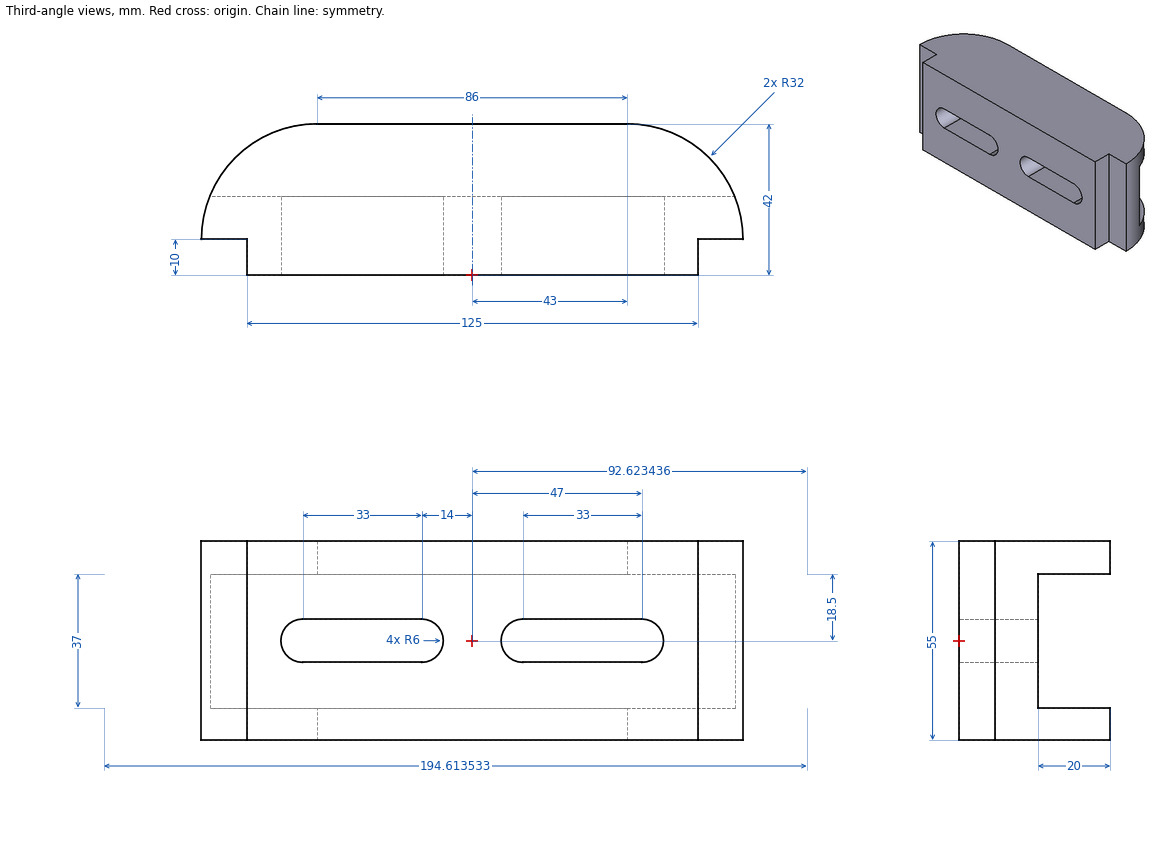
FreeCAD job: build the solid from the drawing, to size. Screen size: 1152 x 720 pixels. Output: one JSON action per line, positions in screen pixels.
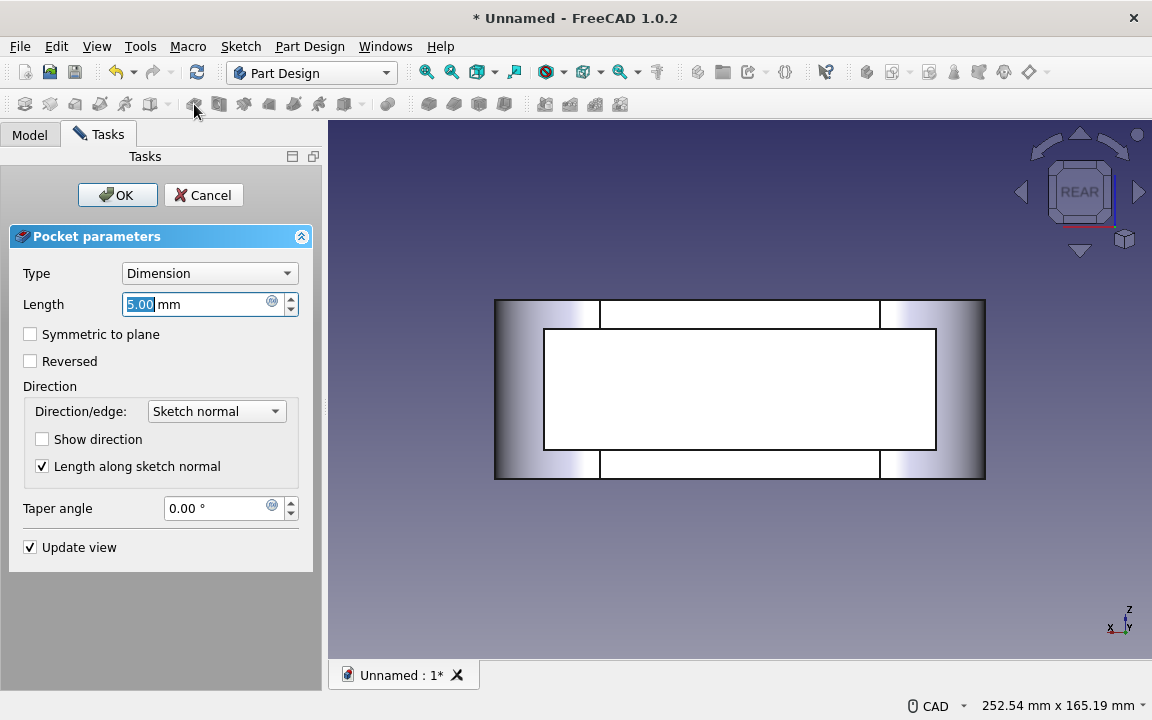
{"action": "type", "text": "20"}
{"action": "key", "text": "Tab"}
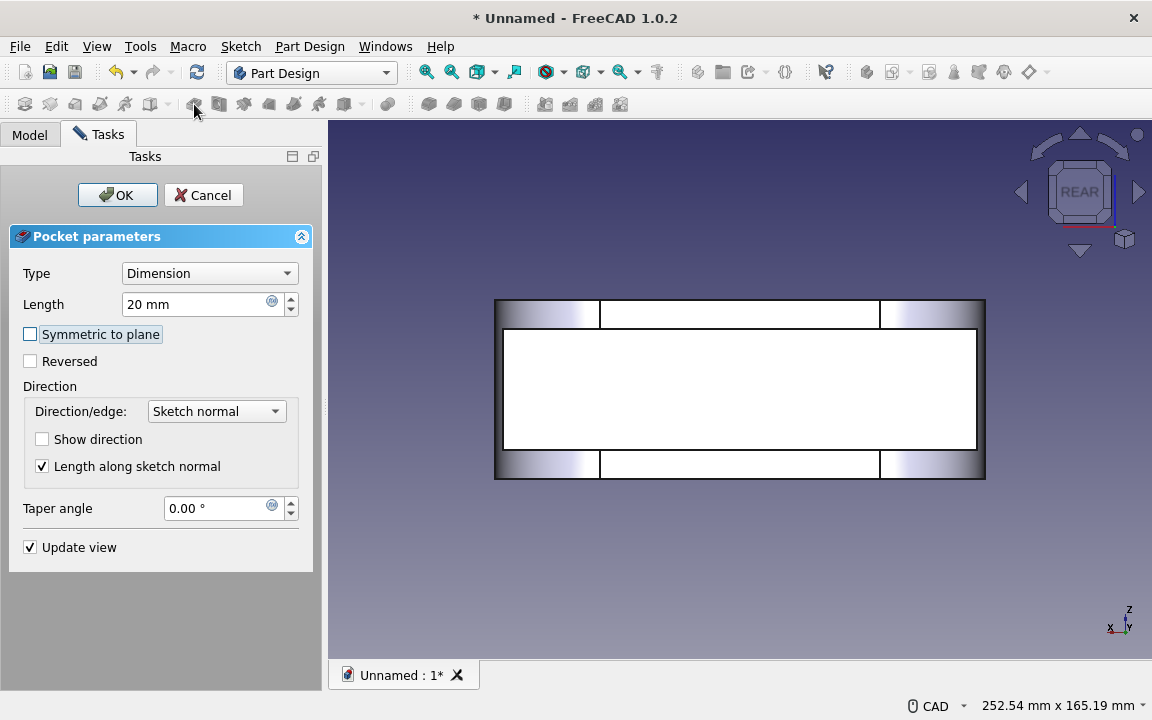
{"action": "left_click", "coordinate": [118, 195]}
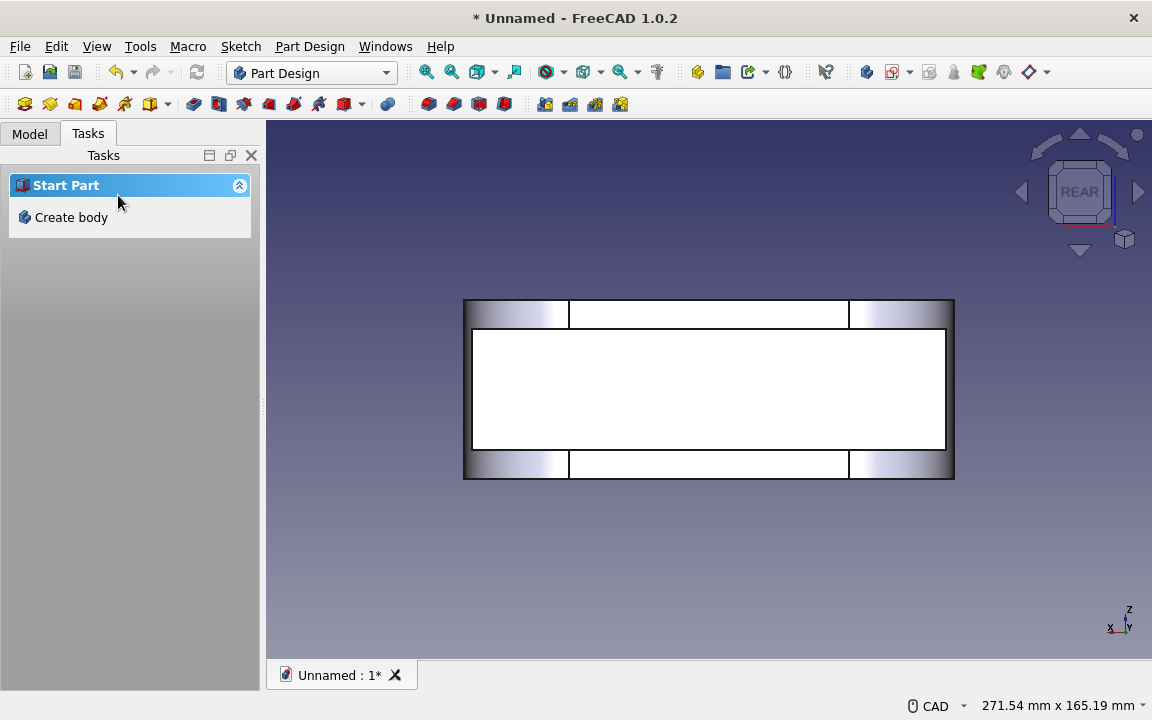
{"action": "left_click", "coordinate": [574, 388]}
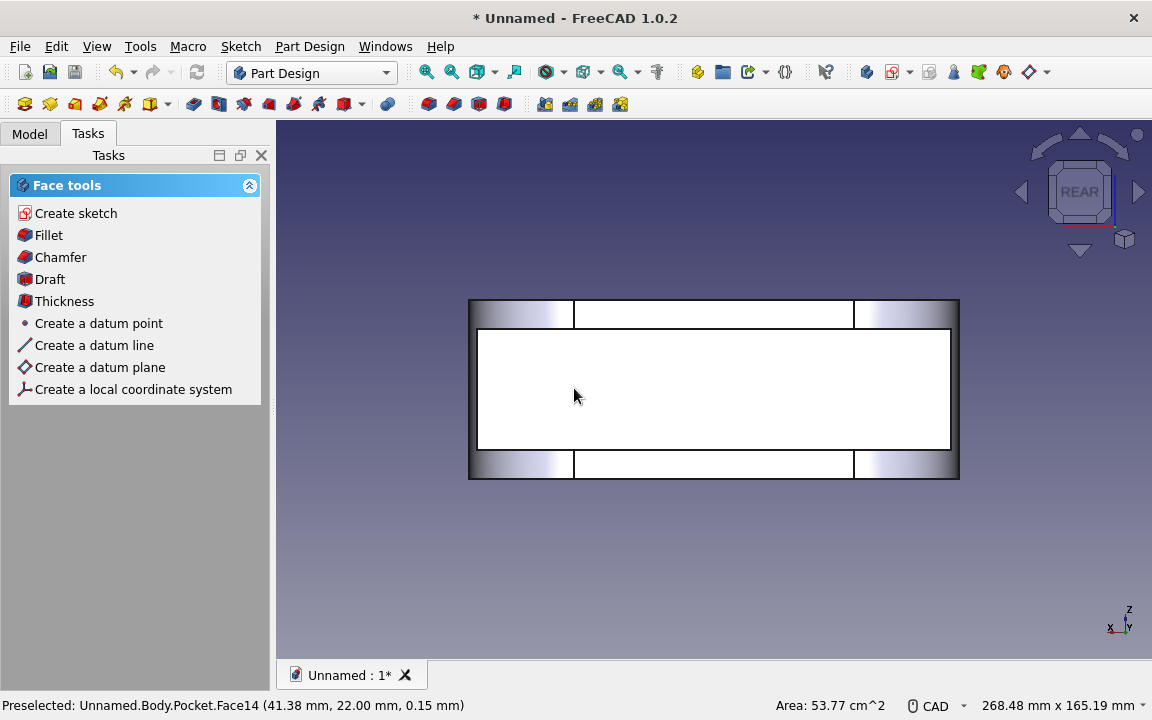
{"action": "left_click", "coordinate": [892, 72]}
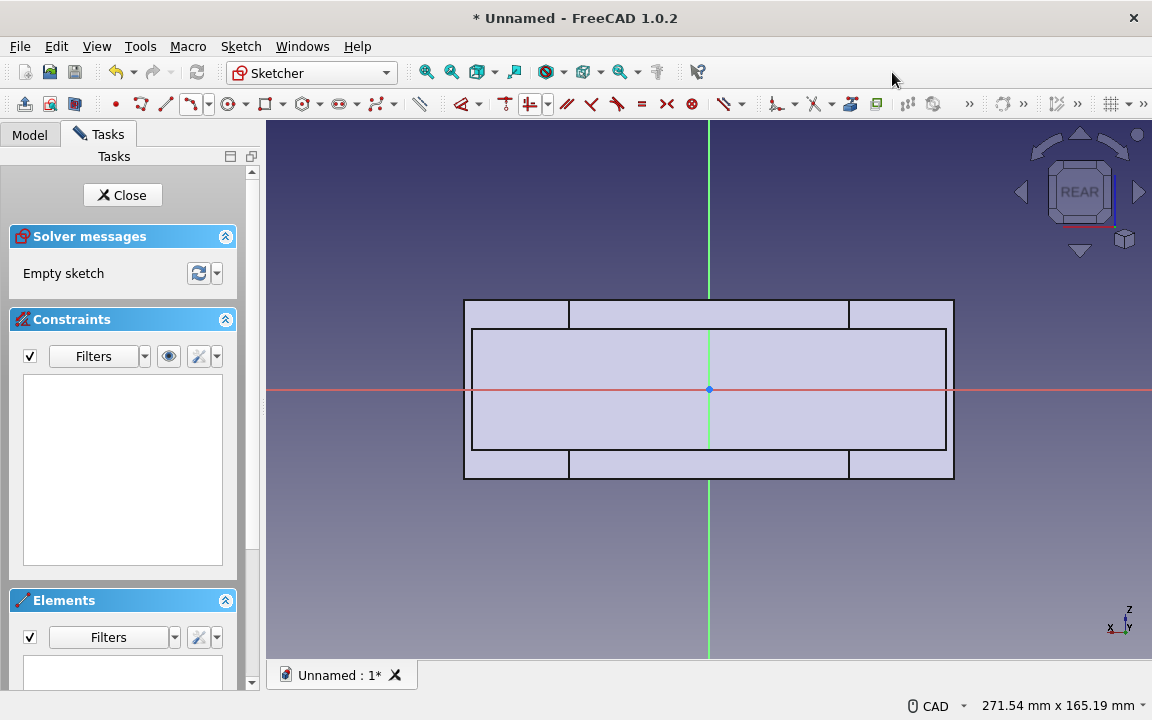
{"action": "left_click", "coordinate": [75, 104]}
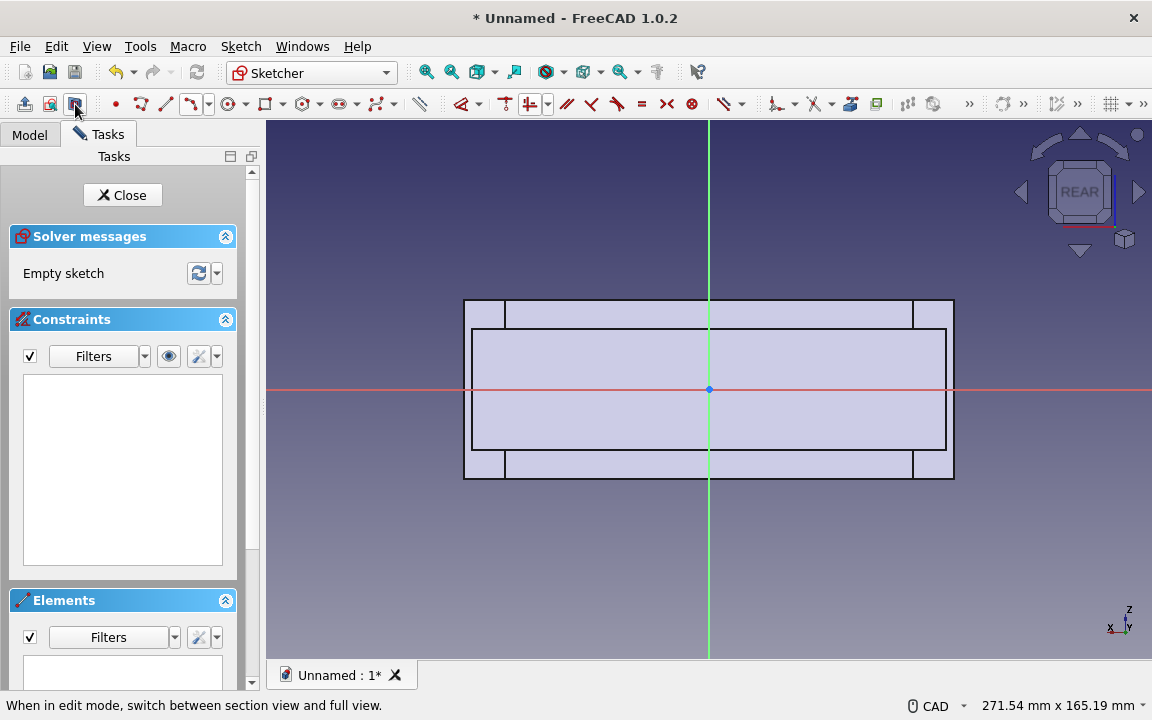
{"action": "scroll", "coordinate": [848, 390], "scroll_direction": "up", "scroll_amount": 2}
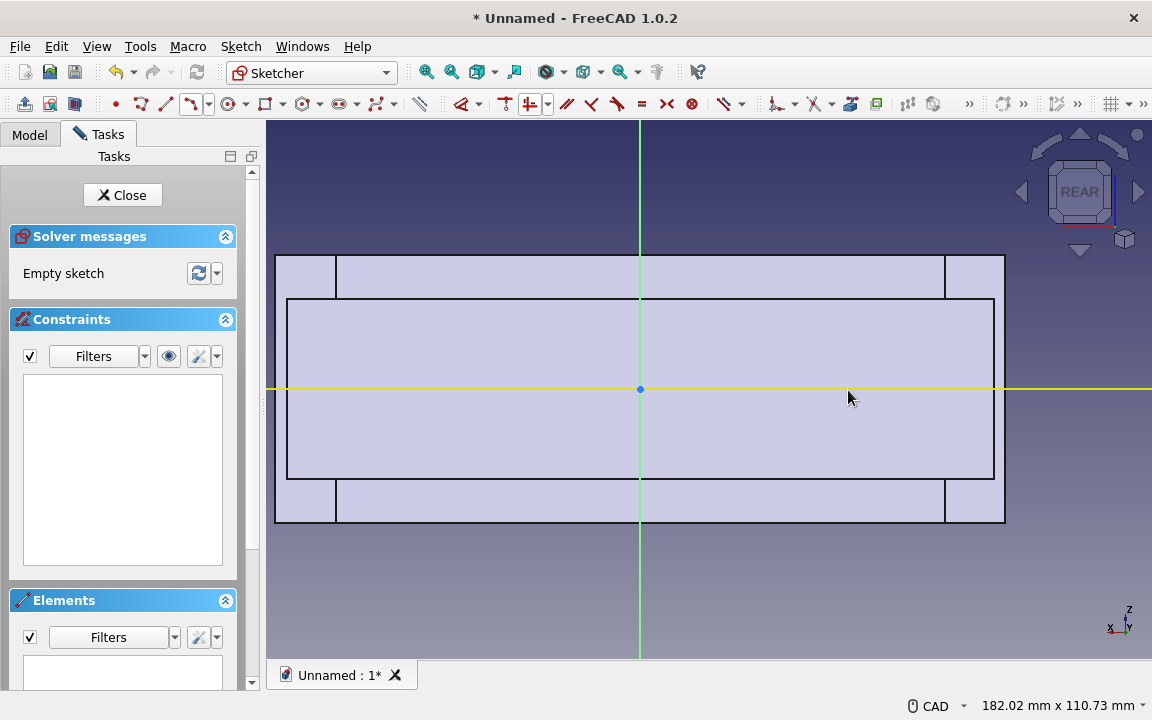
{"action": "left_click", "coordinate": [338, 104]}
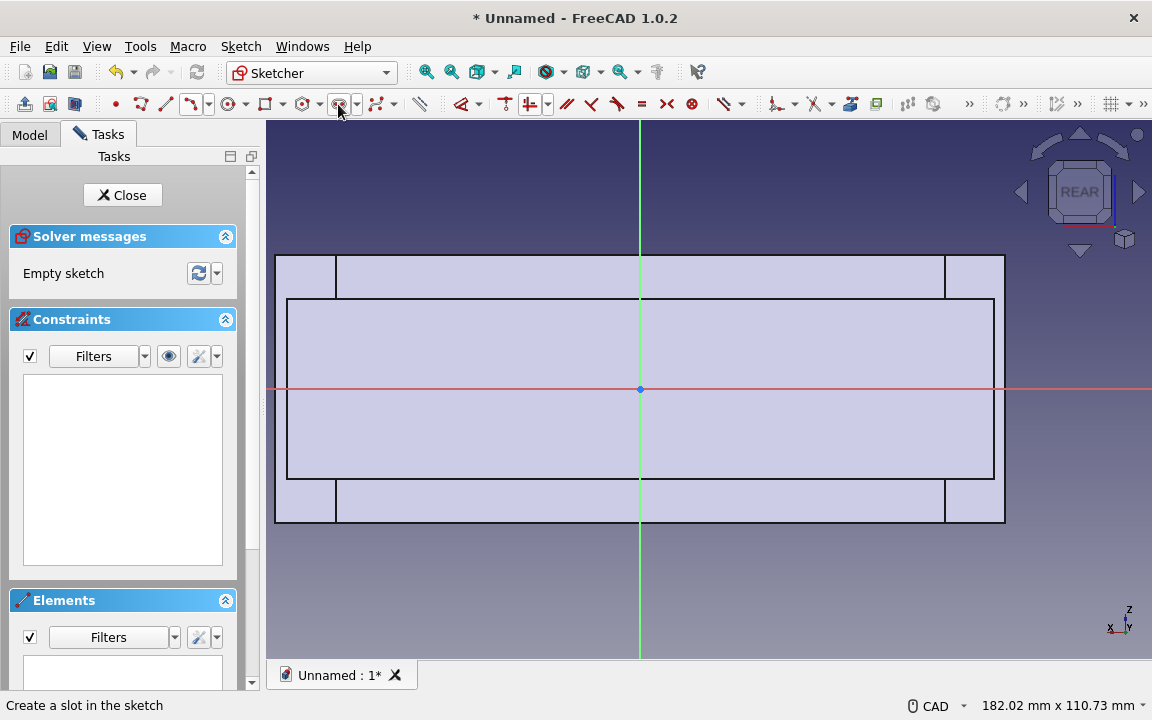
{"action": "left_click", "coordinate": [708, 389]}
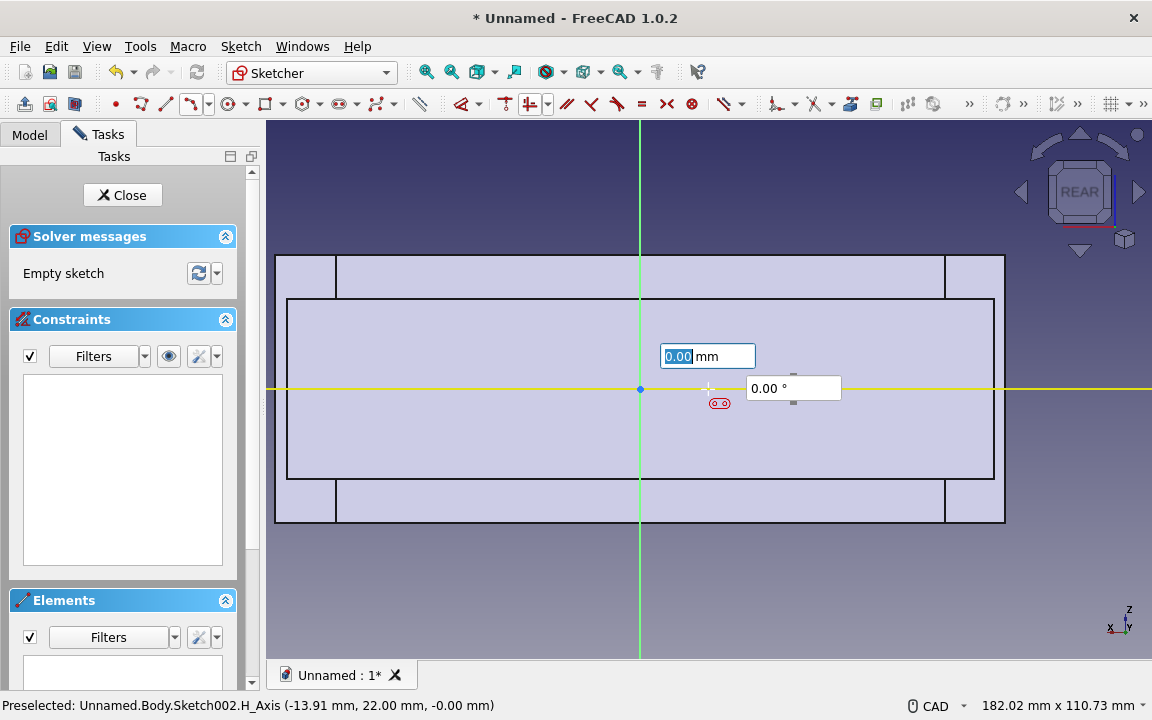
{"action": "left_click", "coordinate": [869, 380]}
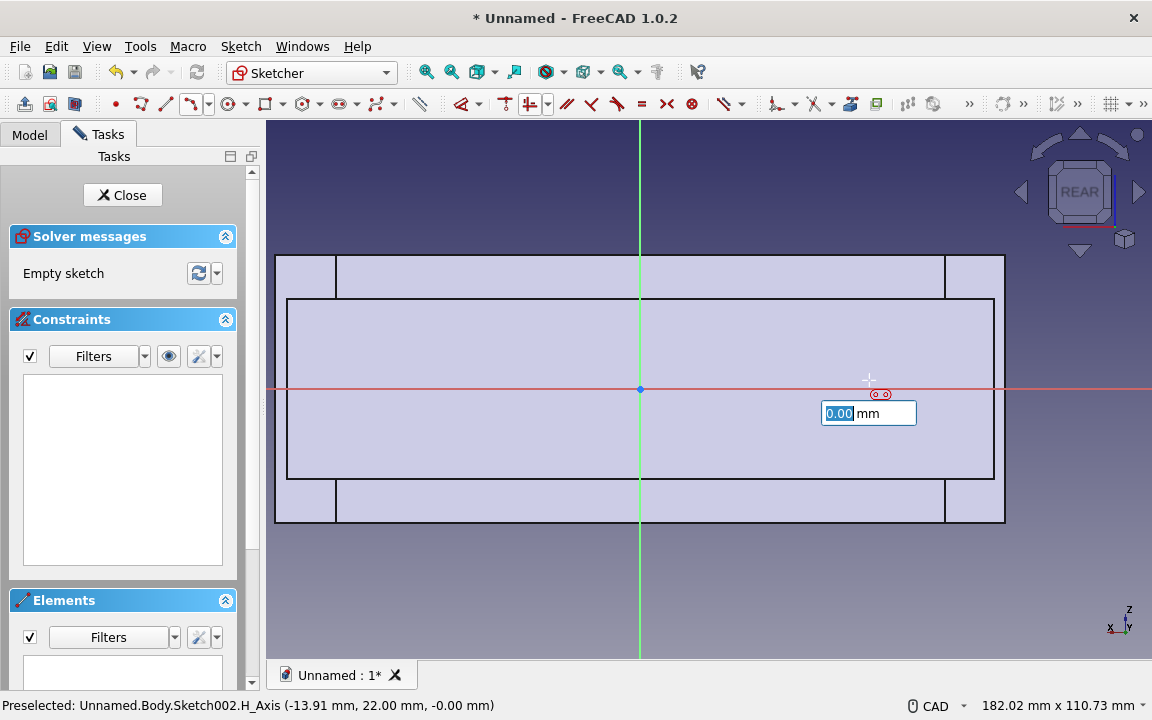
{"action": "left_click", "coordinate": [789, 360]}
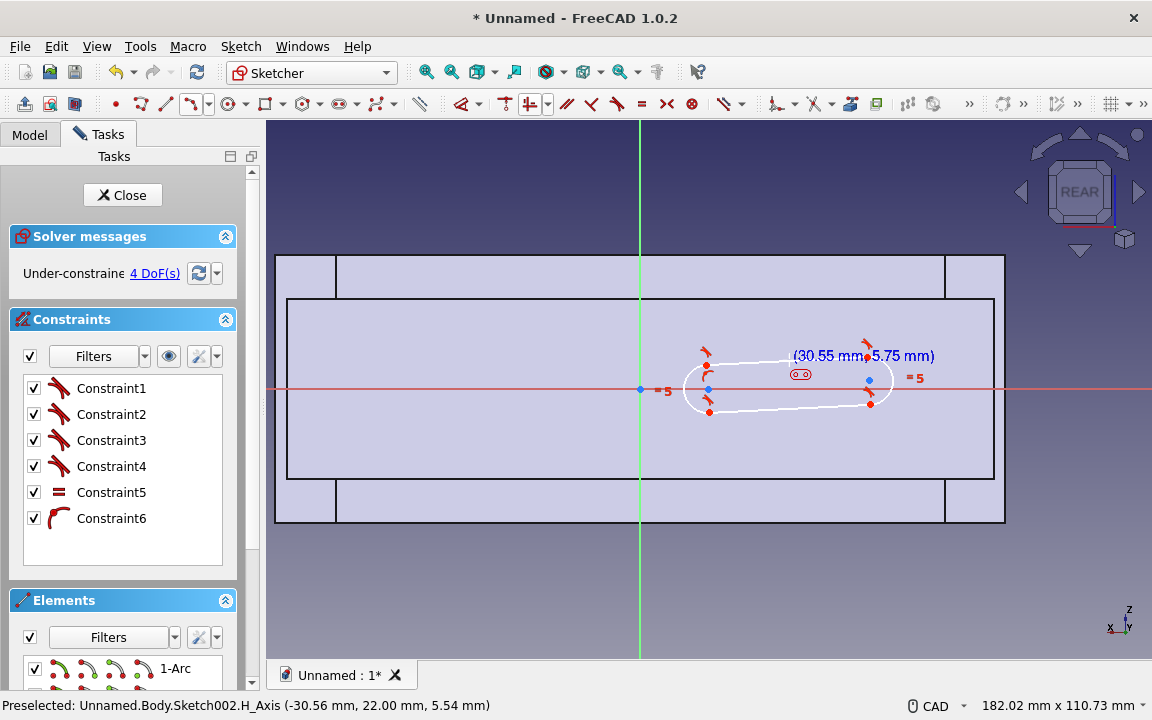
{"action": "left_click", "coordinate": [412, 389]}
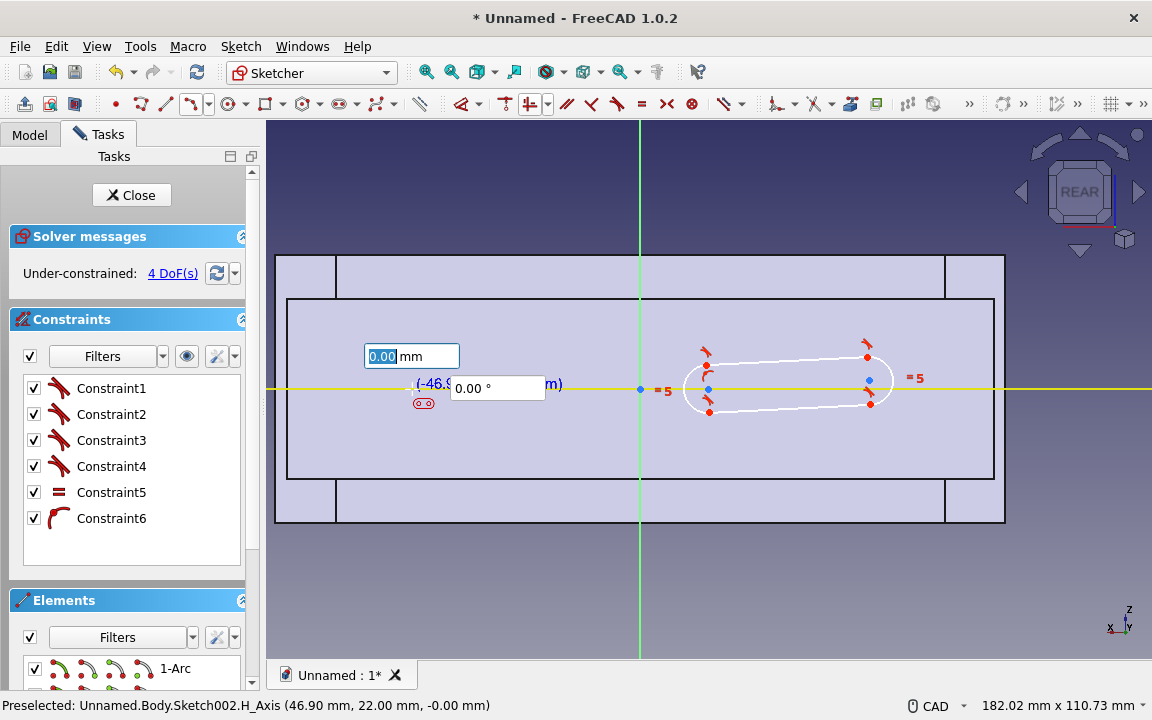
{"action": "left_click", "coordinate": [572, 380]}